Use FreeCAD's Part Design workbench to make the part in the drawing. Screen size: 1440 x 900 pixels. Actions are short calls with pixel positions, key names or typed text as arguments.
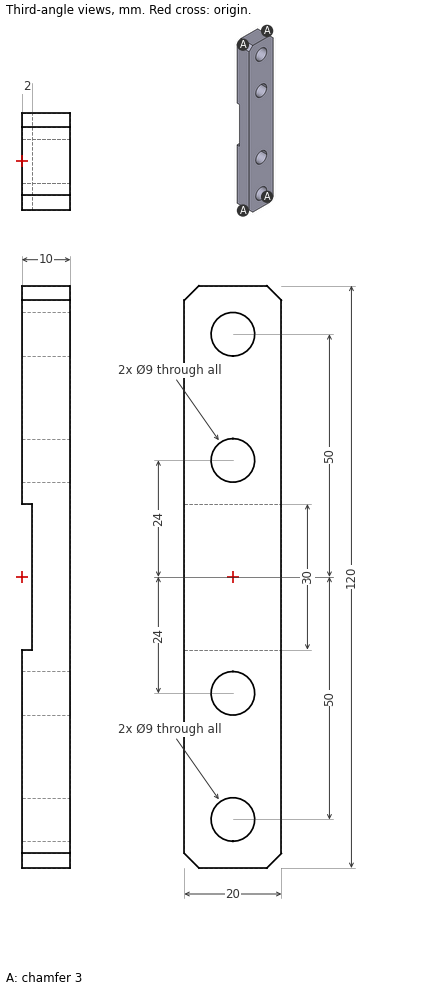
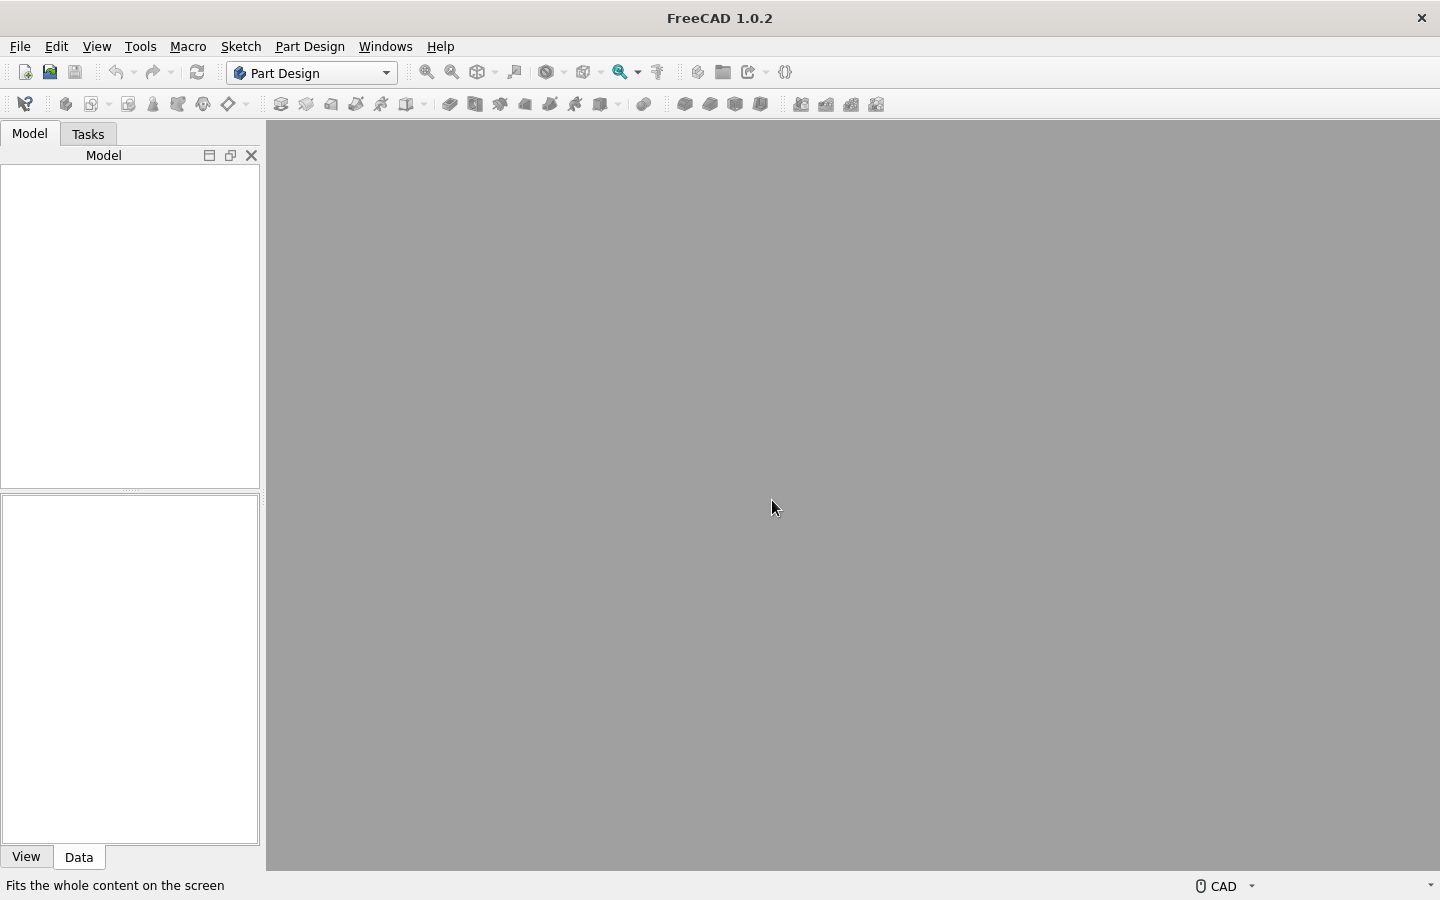
key(ctrl+n)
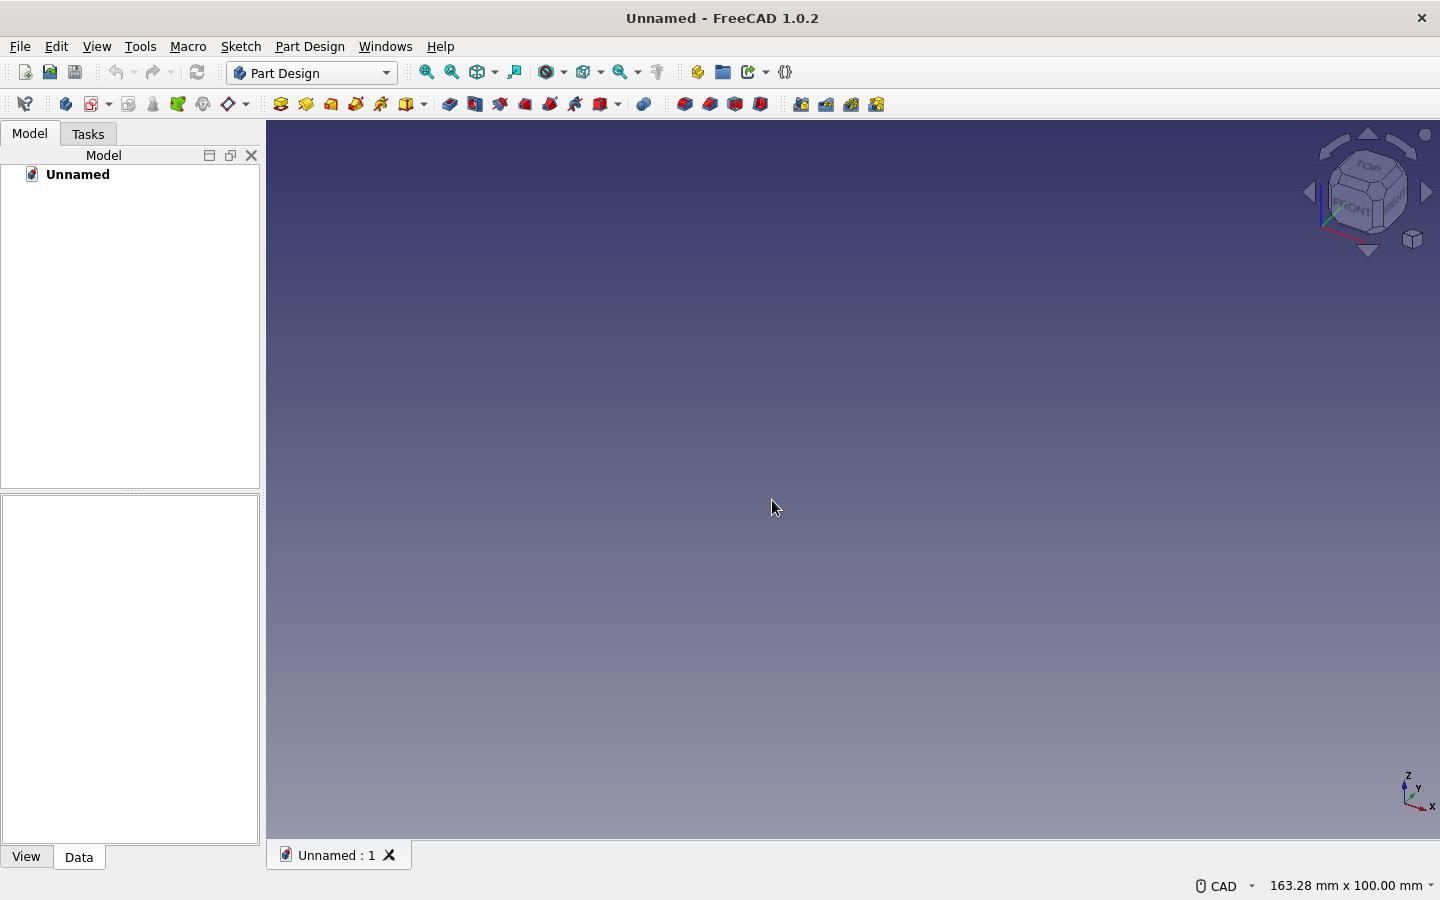
click(90, 104)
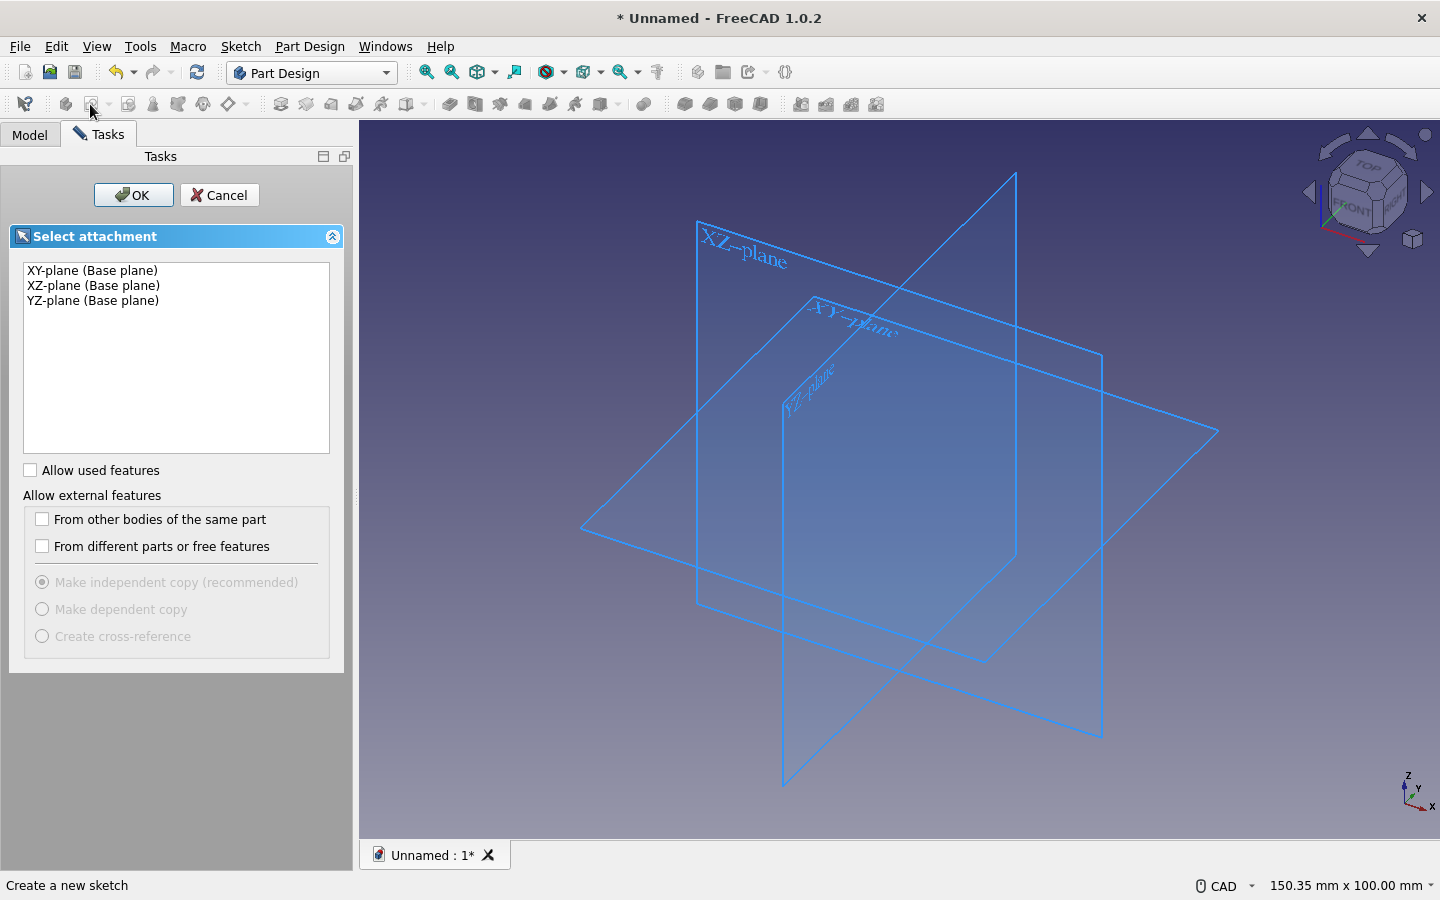
click(84, 300)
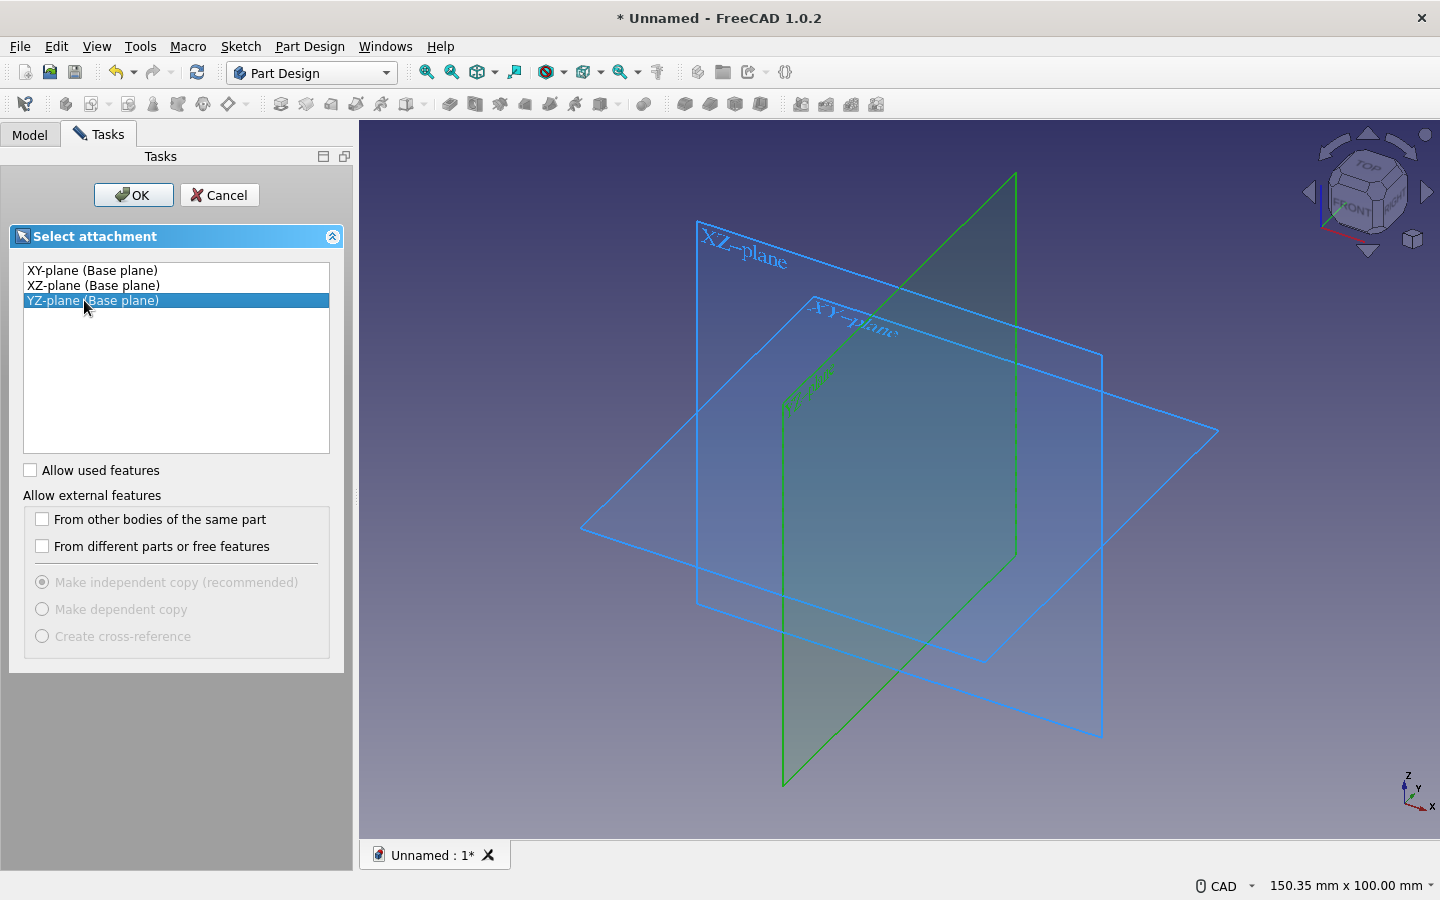
click(134, 195)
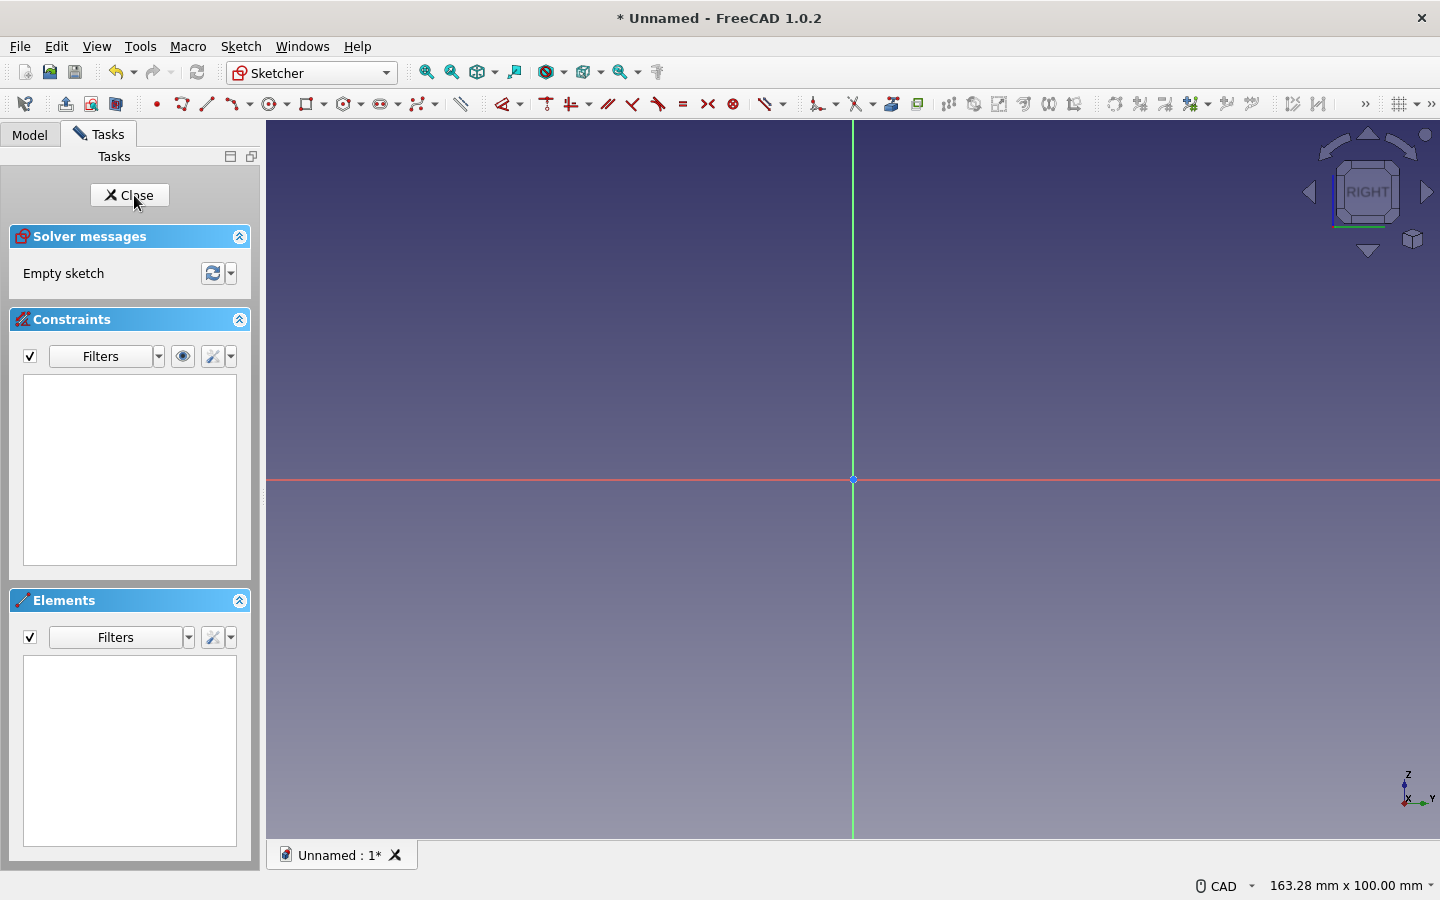
scroll(701, 479, down, 3)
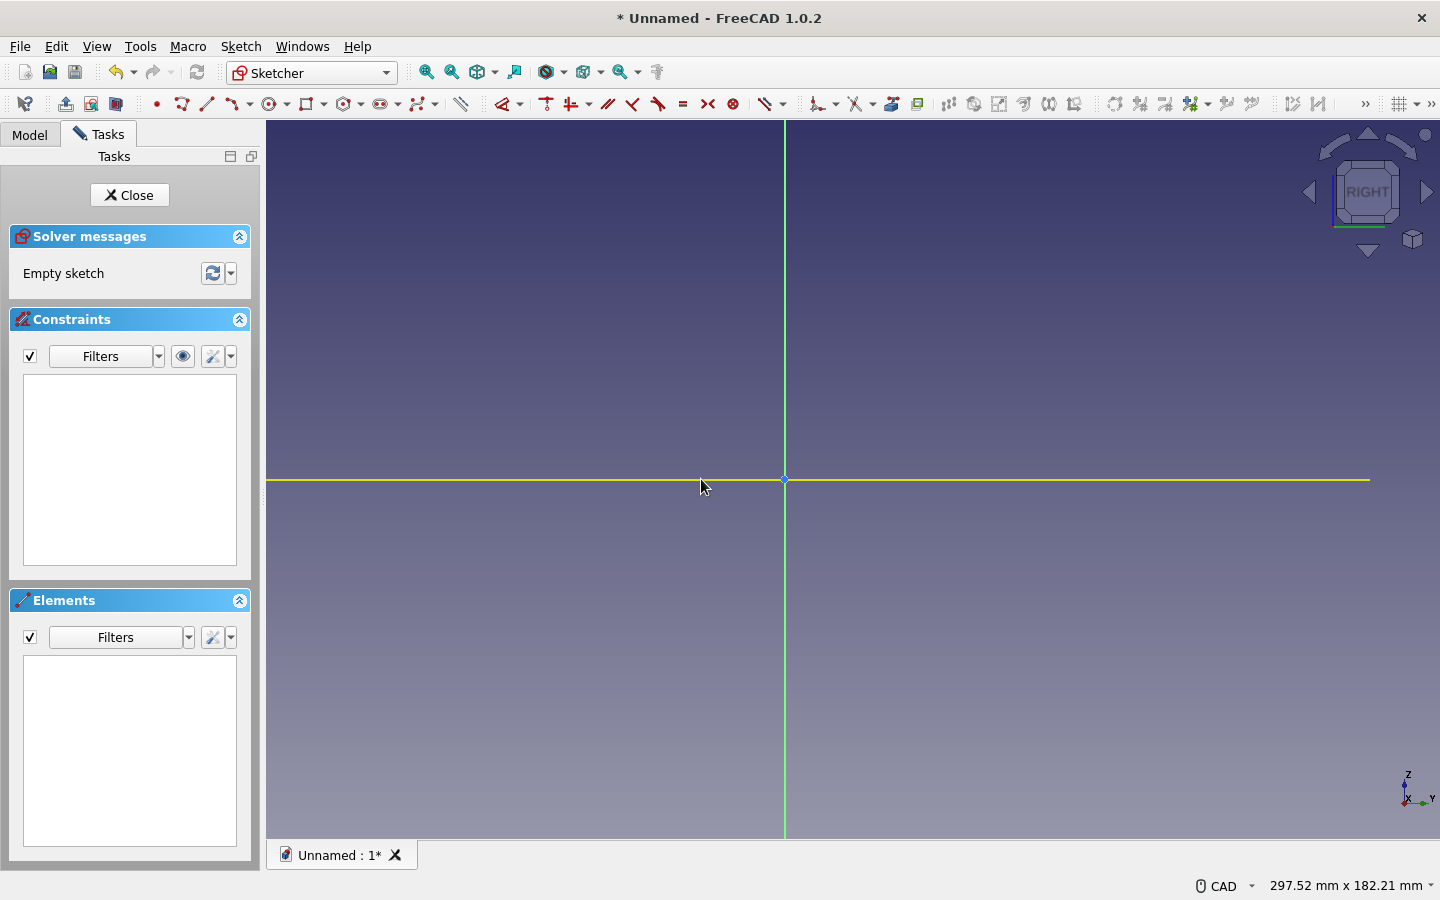
key(g)
key(v)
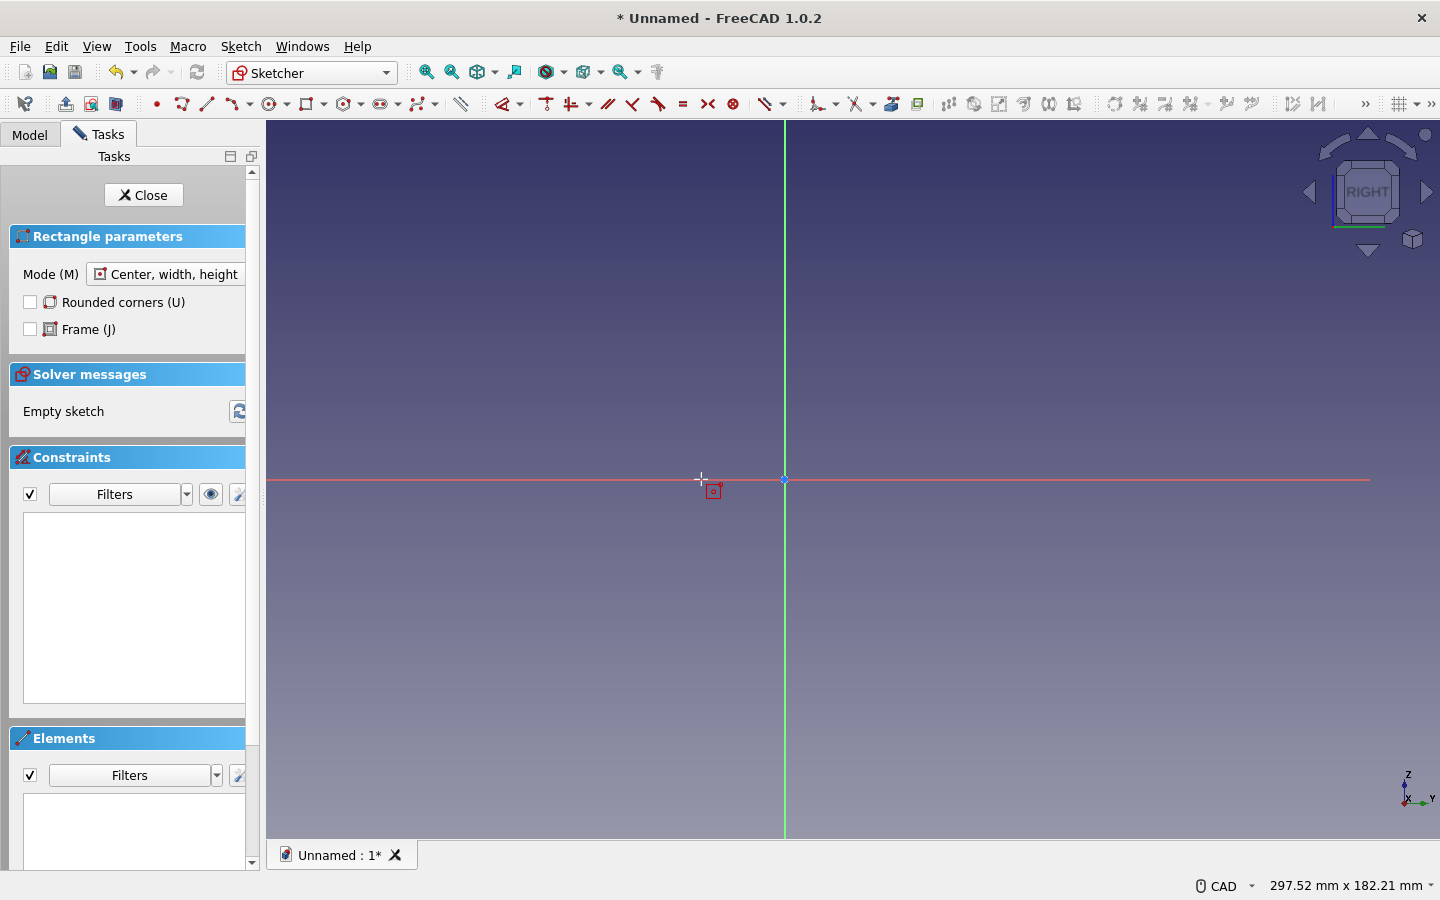
click(785, 480)
move(824, 243)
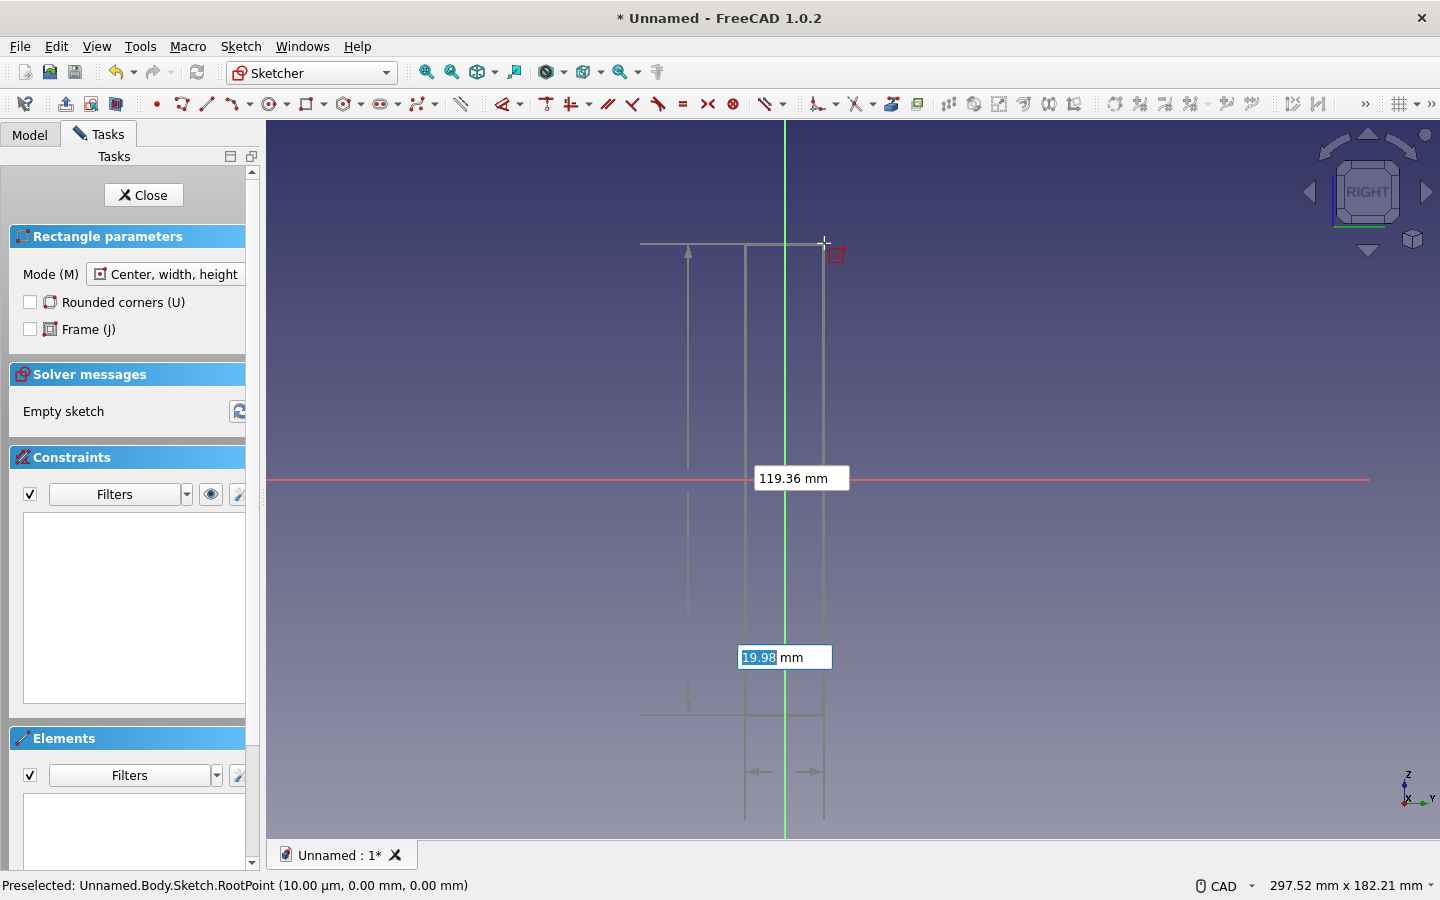
text(20)
key(Tab)
text(120)
key(Return)
key(Escape)